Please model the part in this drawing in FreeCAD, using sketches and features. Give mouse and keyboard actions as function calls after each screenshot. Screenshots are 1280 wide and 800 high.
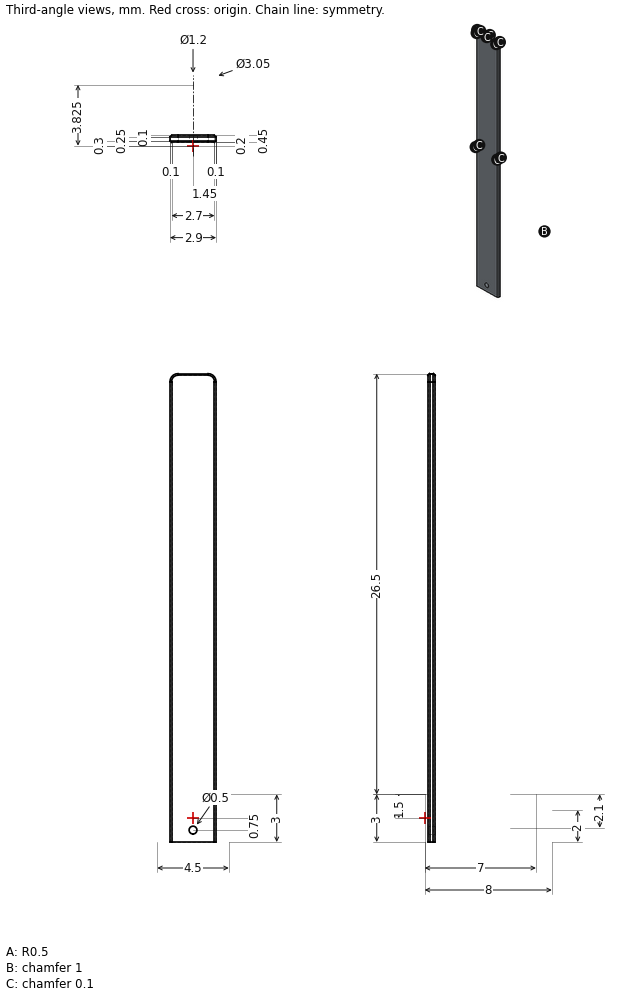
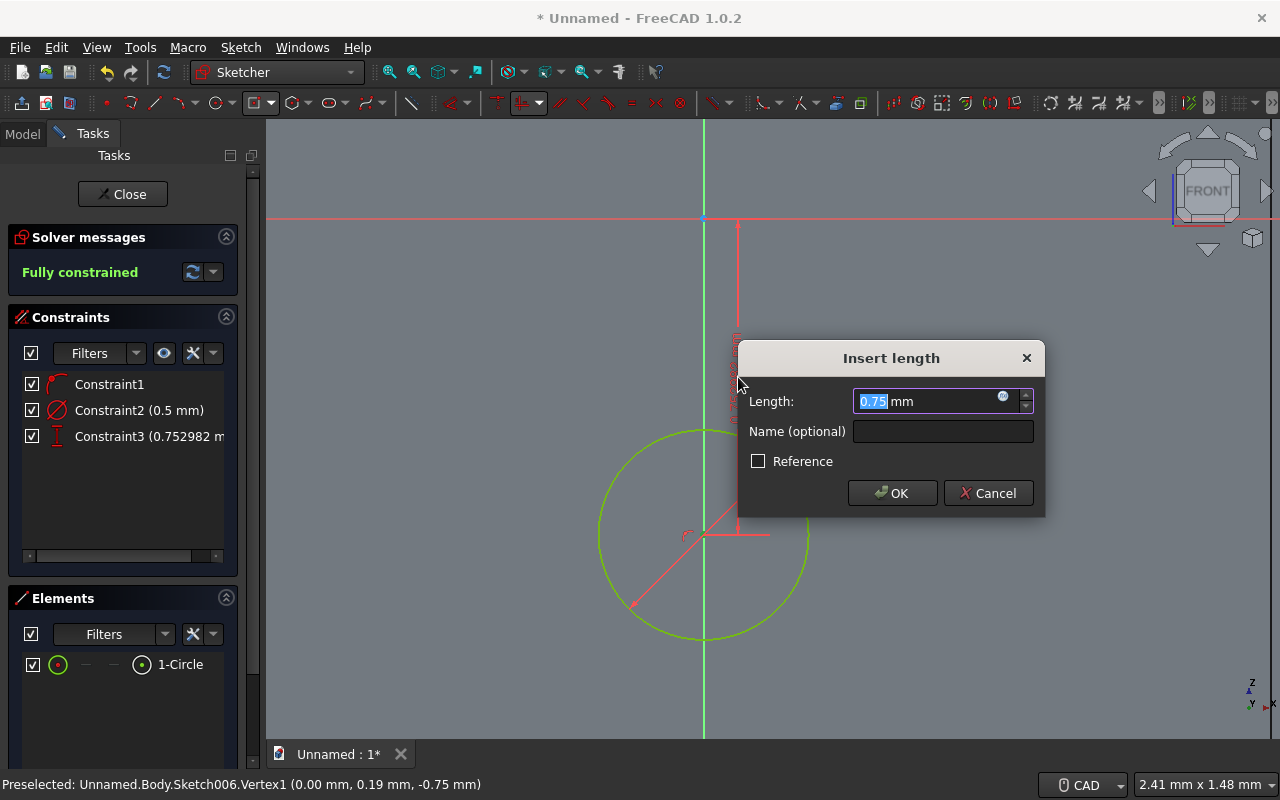
text(0.75)
key(Return)
key(Escape)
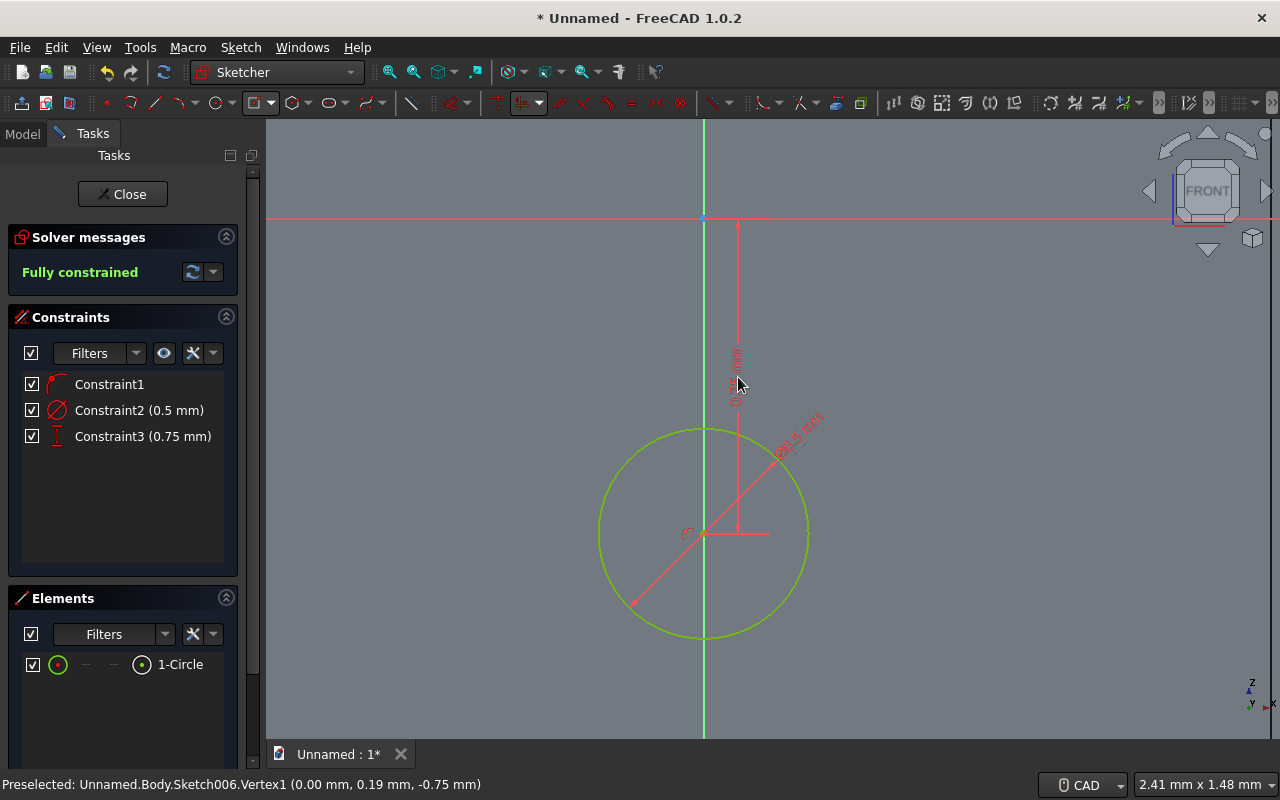
click(123, 194)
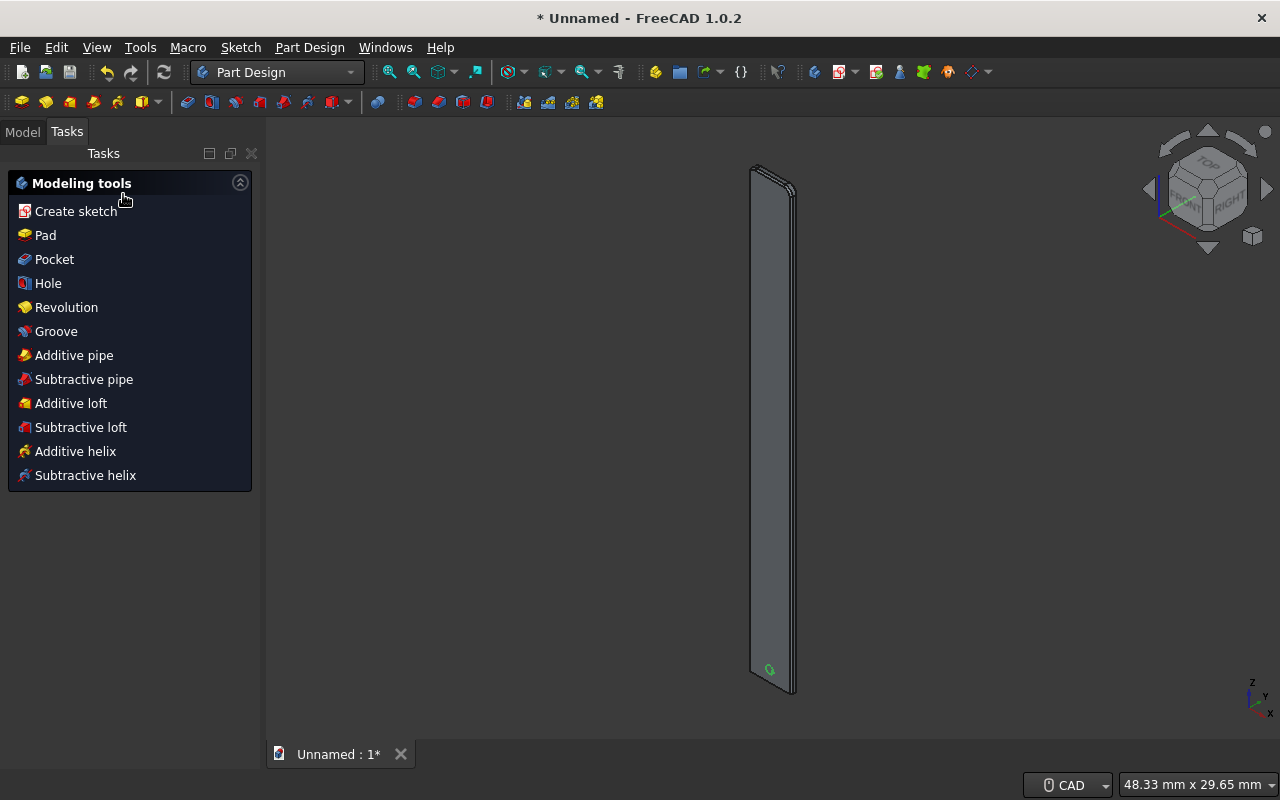
click(188, 102)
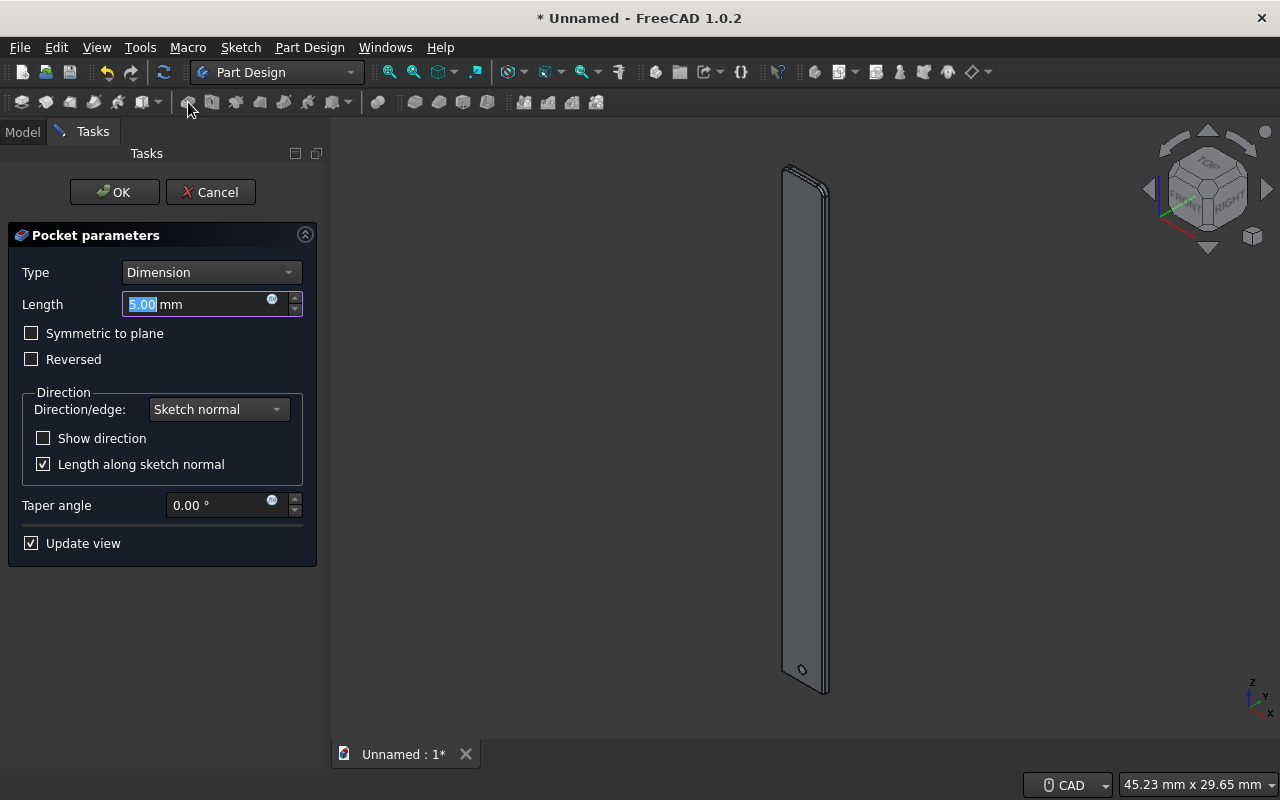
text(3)
key(Tab)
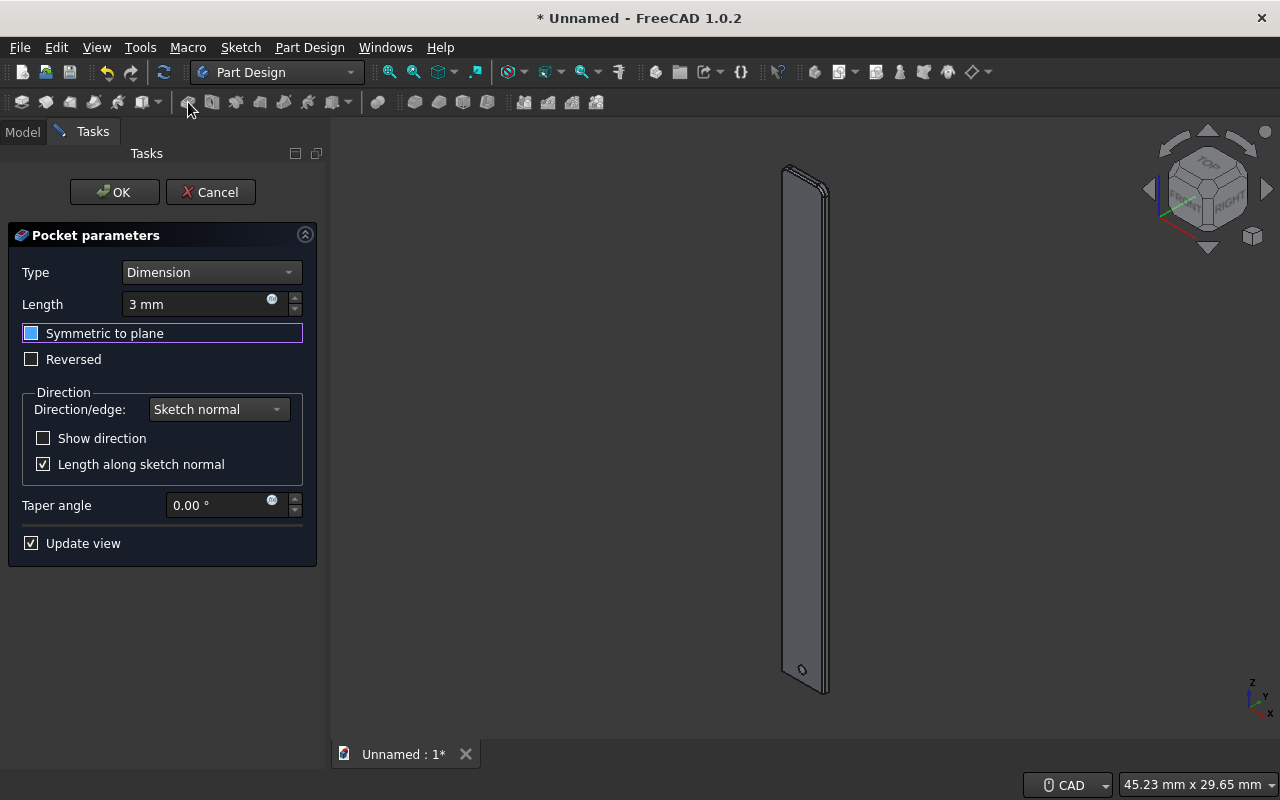
click(115, 192)